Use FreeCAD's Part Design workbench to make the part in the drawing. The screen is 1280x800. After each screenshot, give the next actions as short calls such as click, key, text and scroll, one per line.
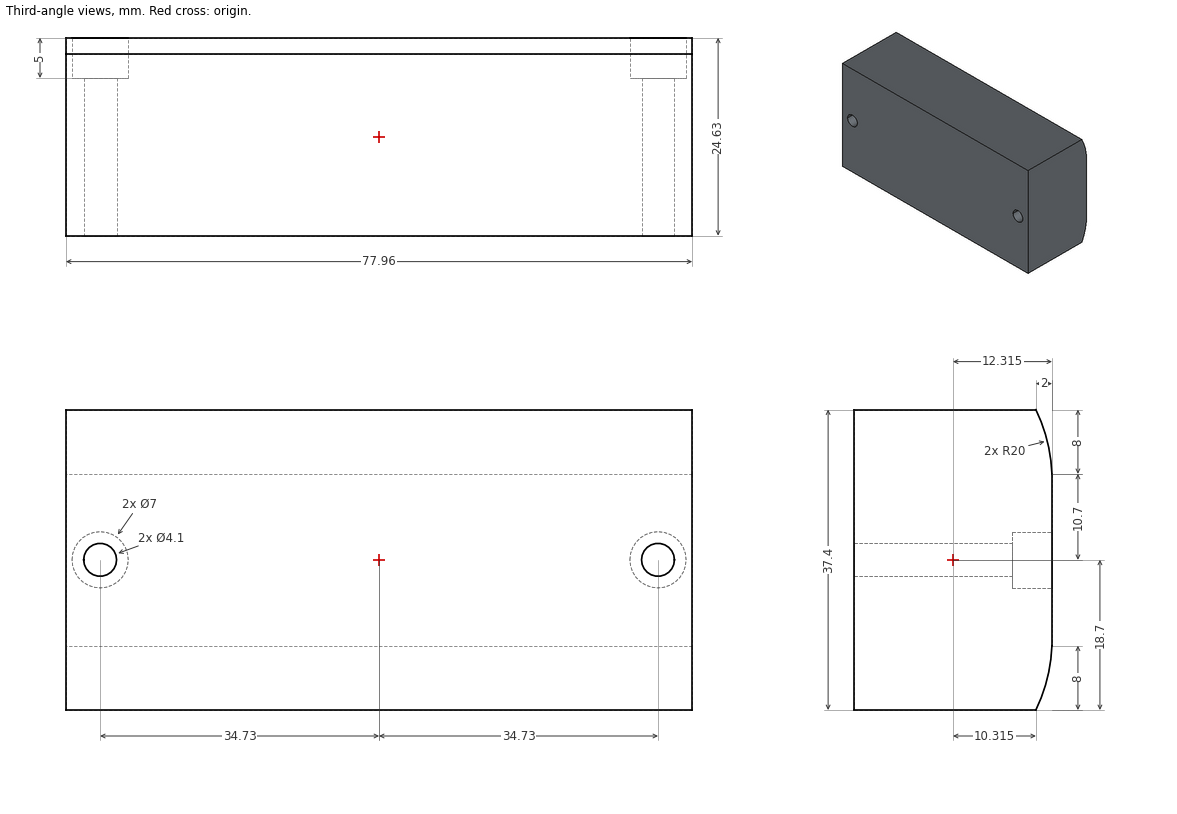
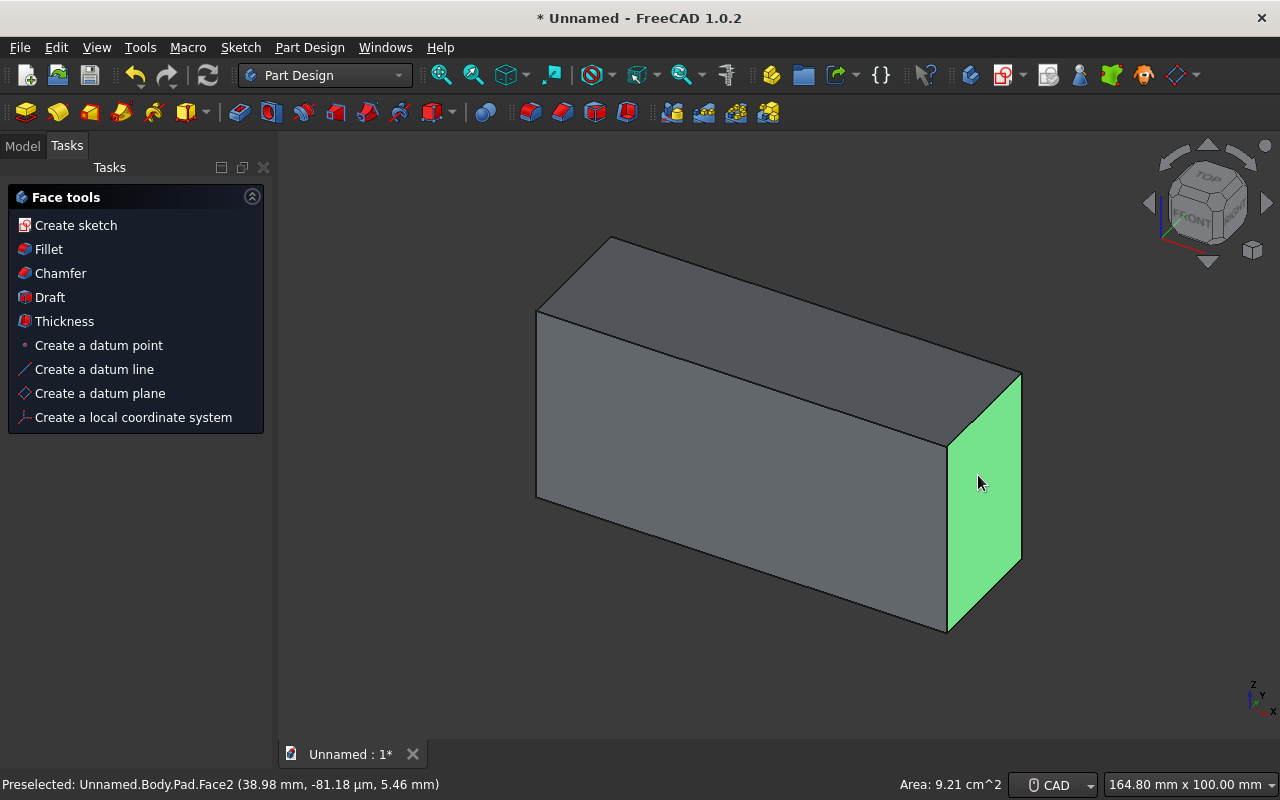
click(1004, 76)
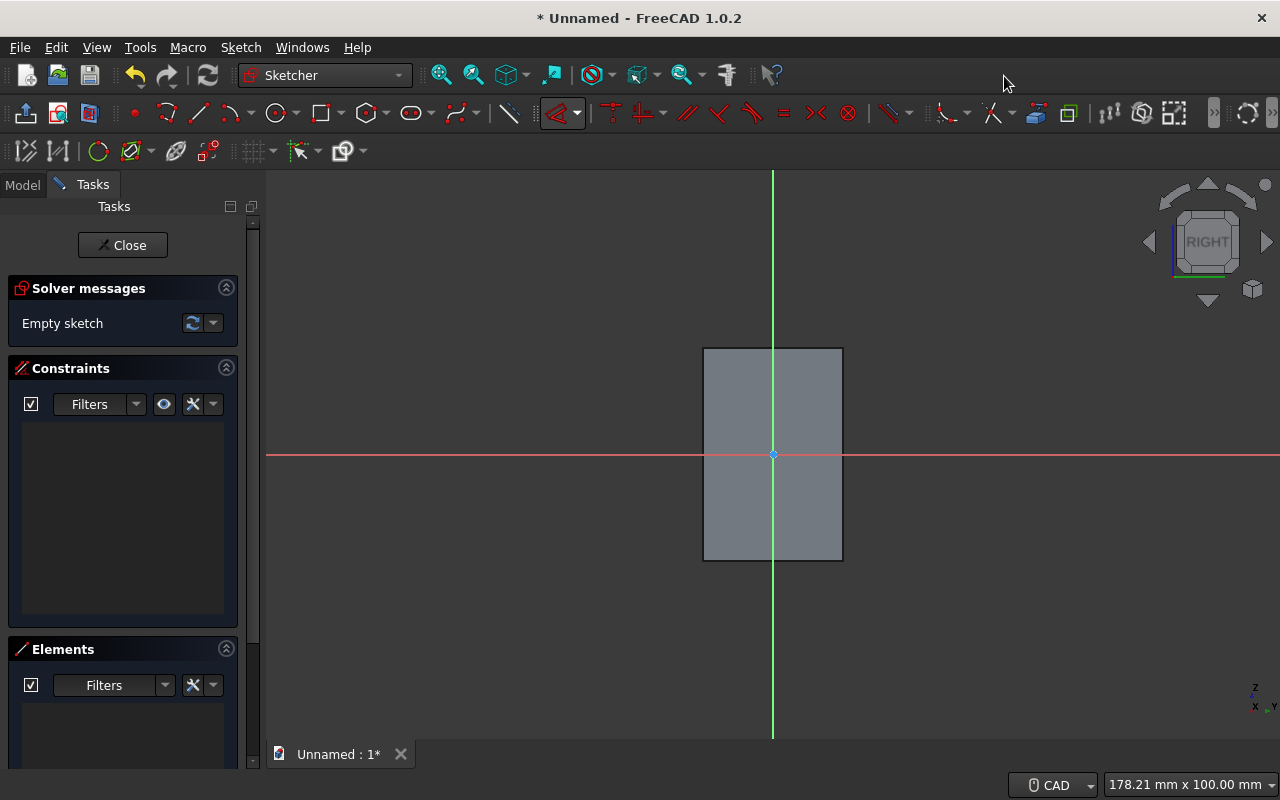
scroll(934, 454, up, 3)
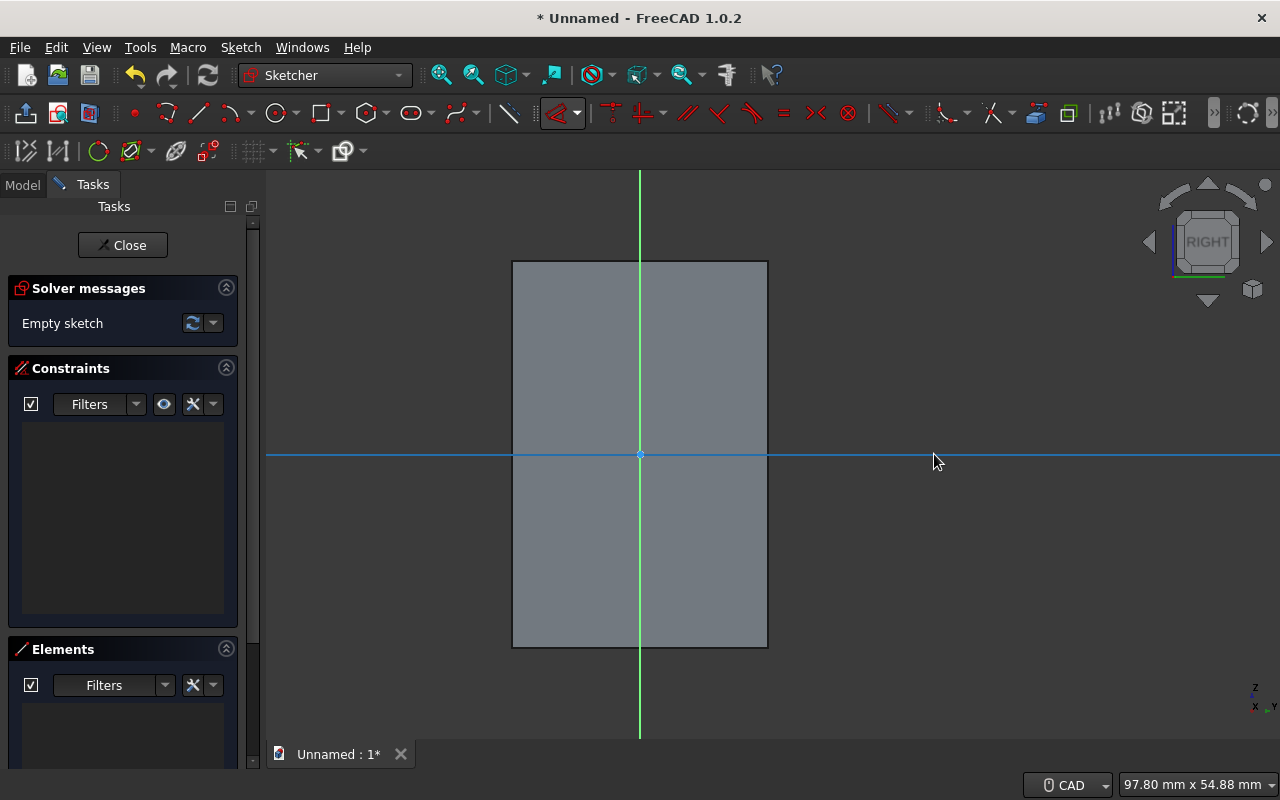
click(168, 114)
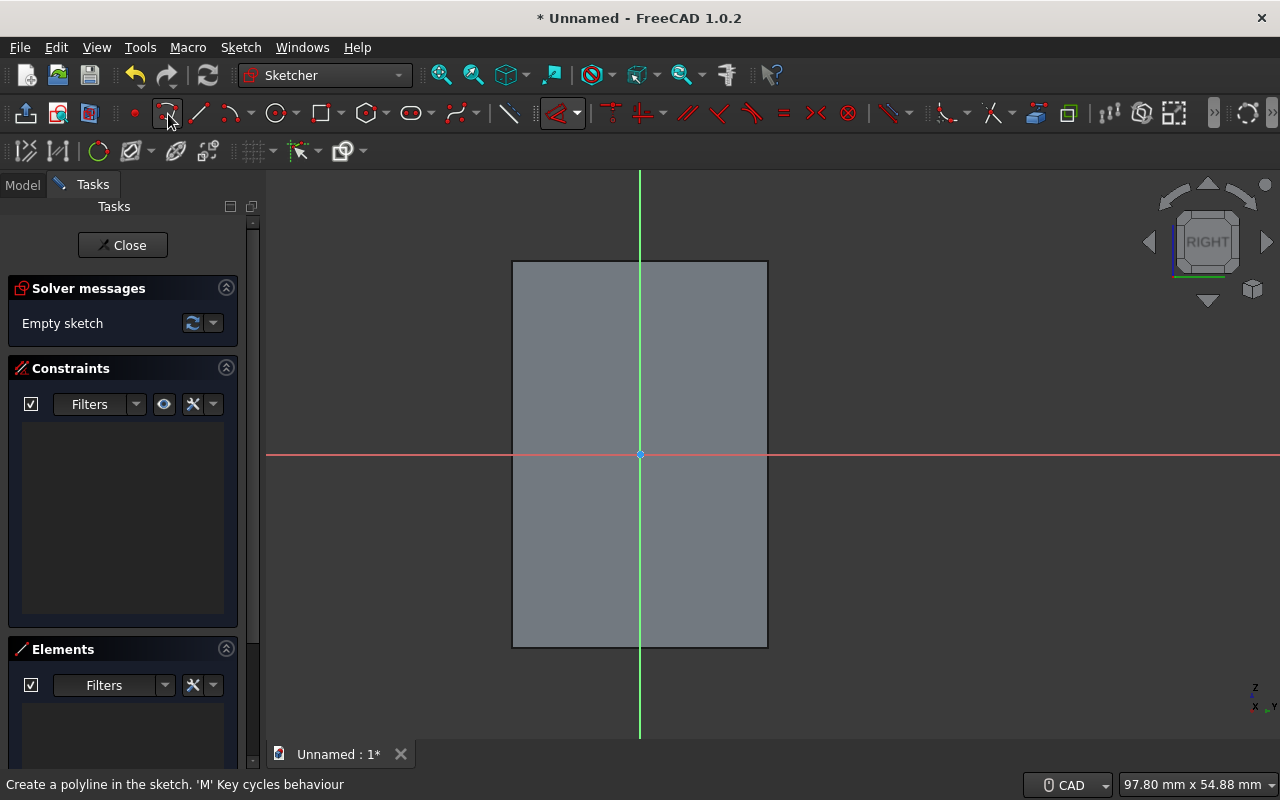
click(768, 344)
click(768, 261)
click(747, 261)
right_click(747, 261)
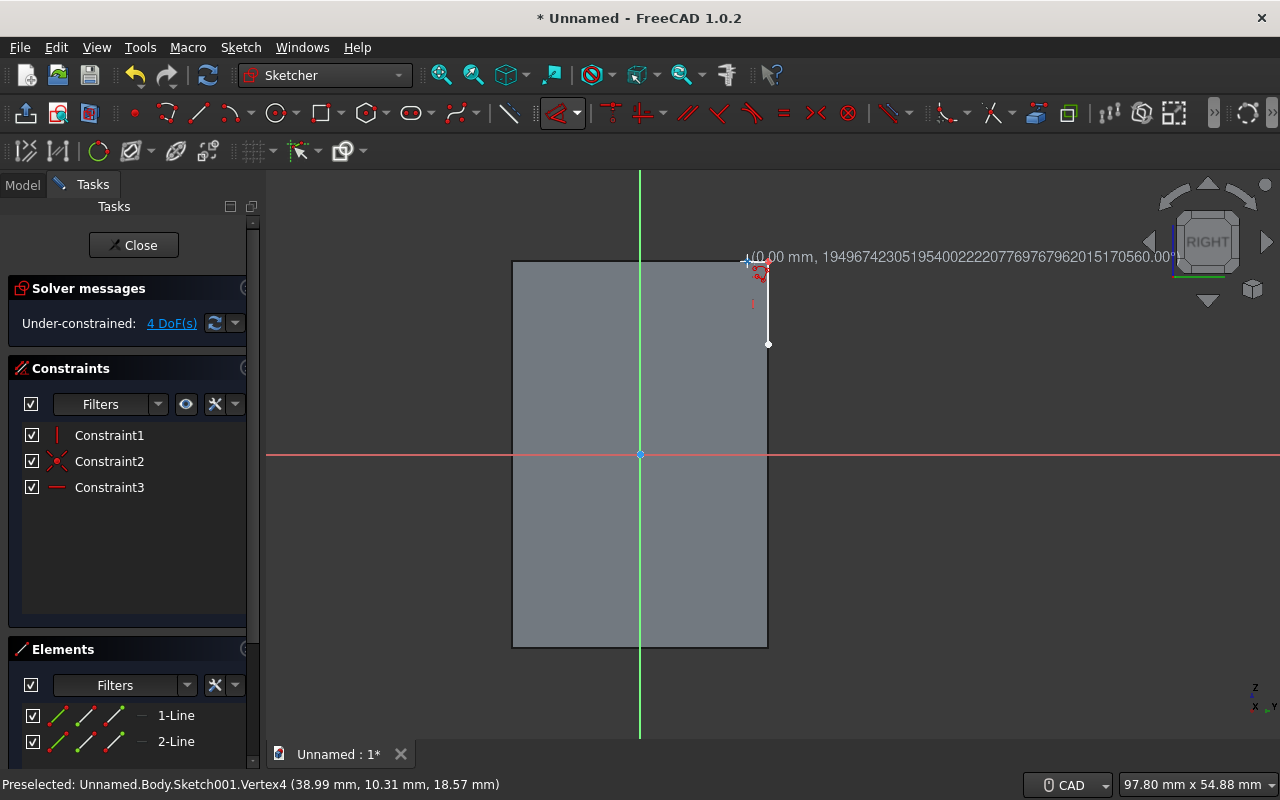
click(254, 114)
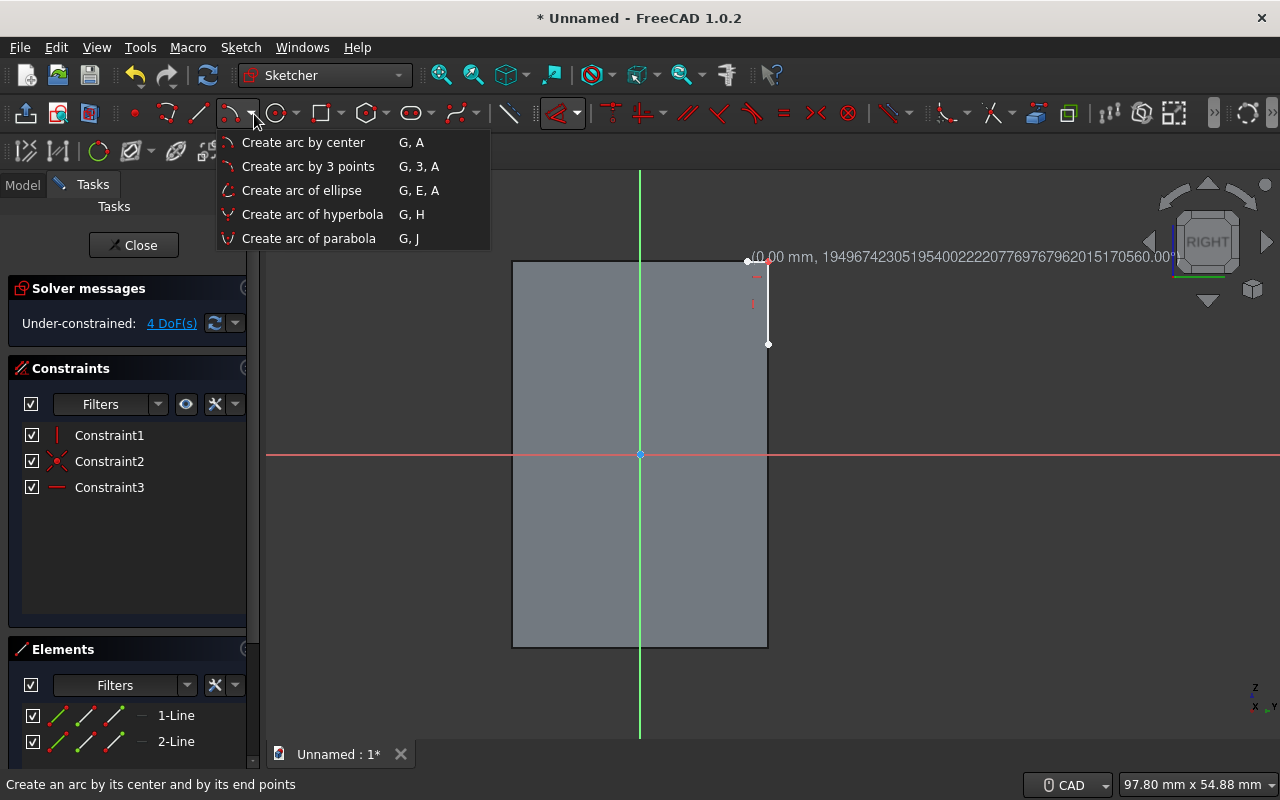
click(354, 166)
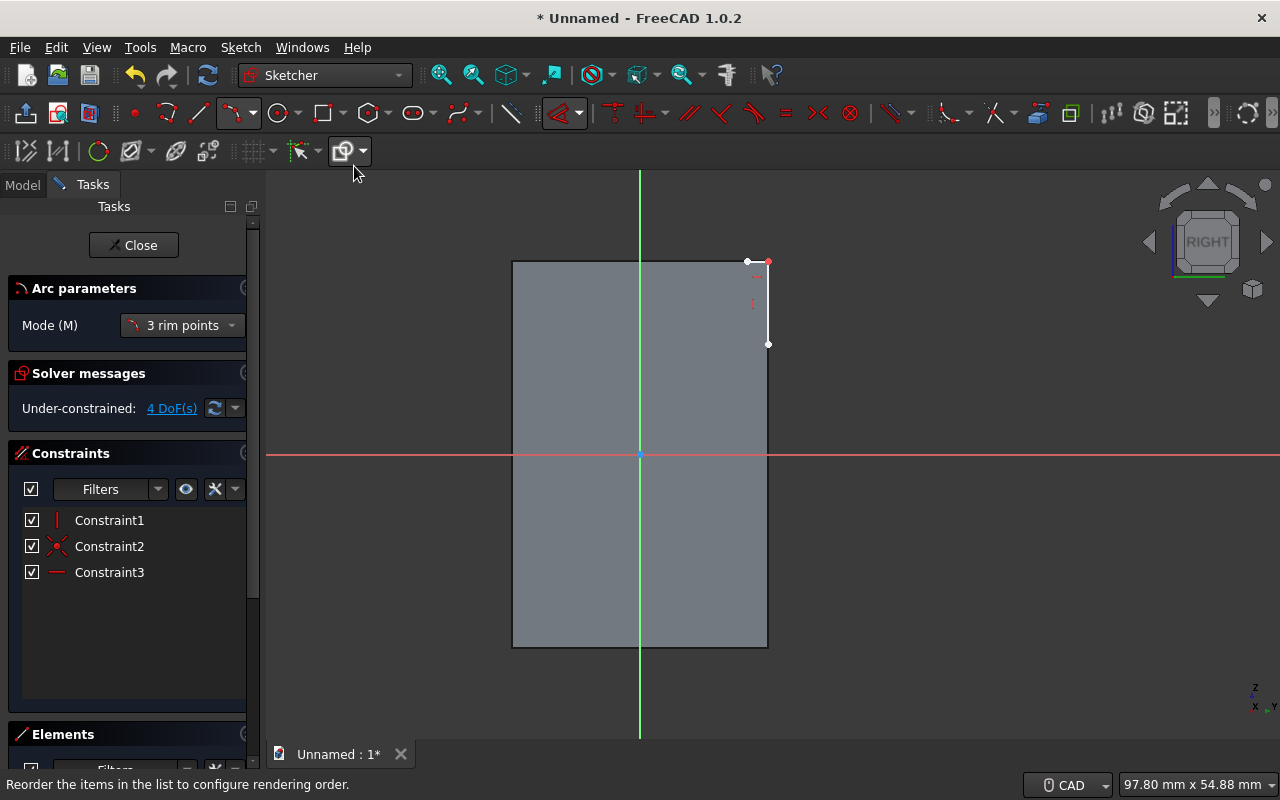
scroll(747, 261, up, 3)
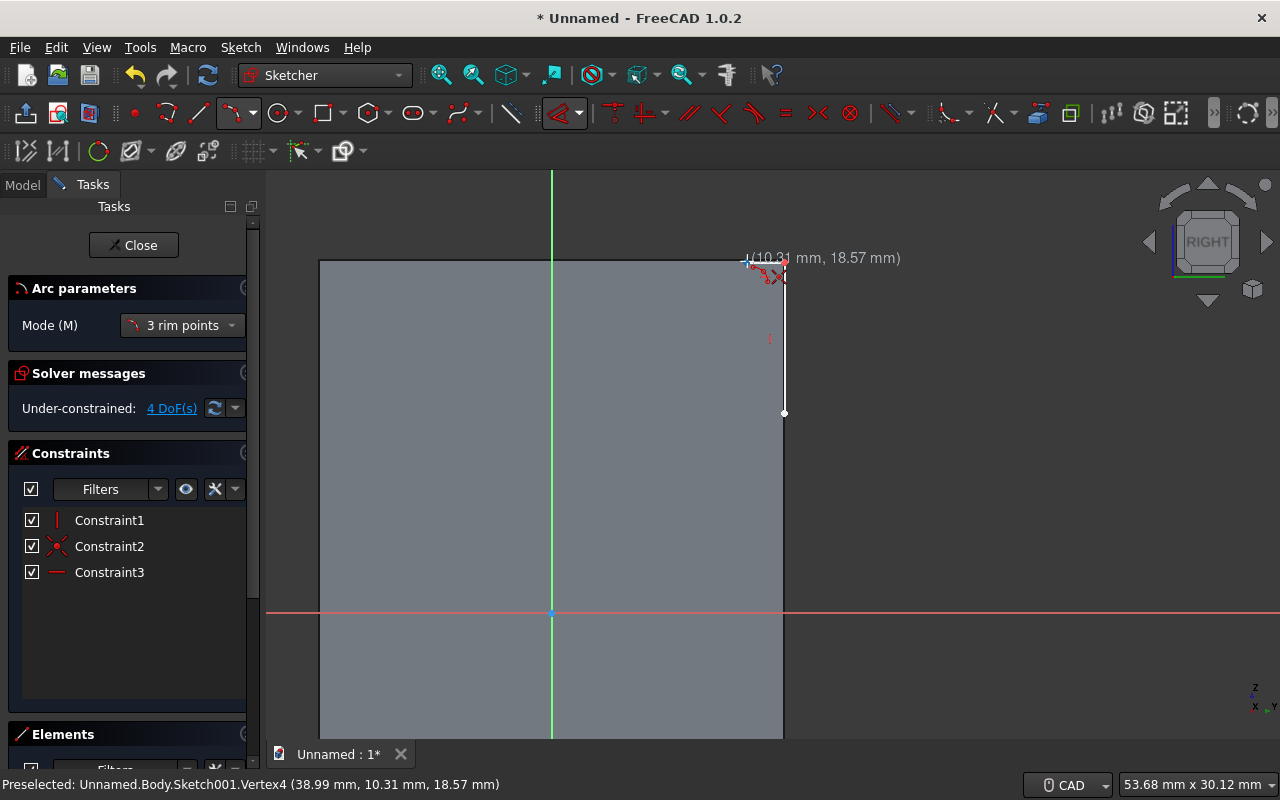
click(747, 263)
click(785, 414)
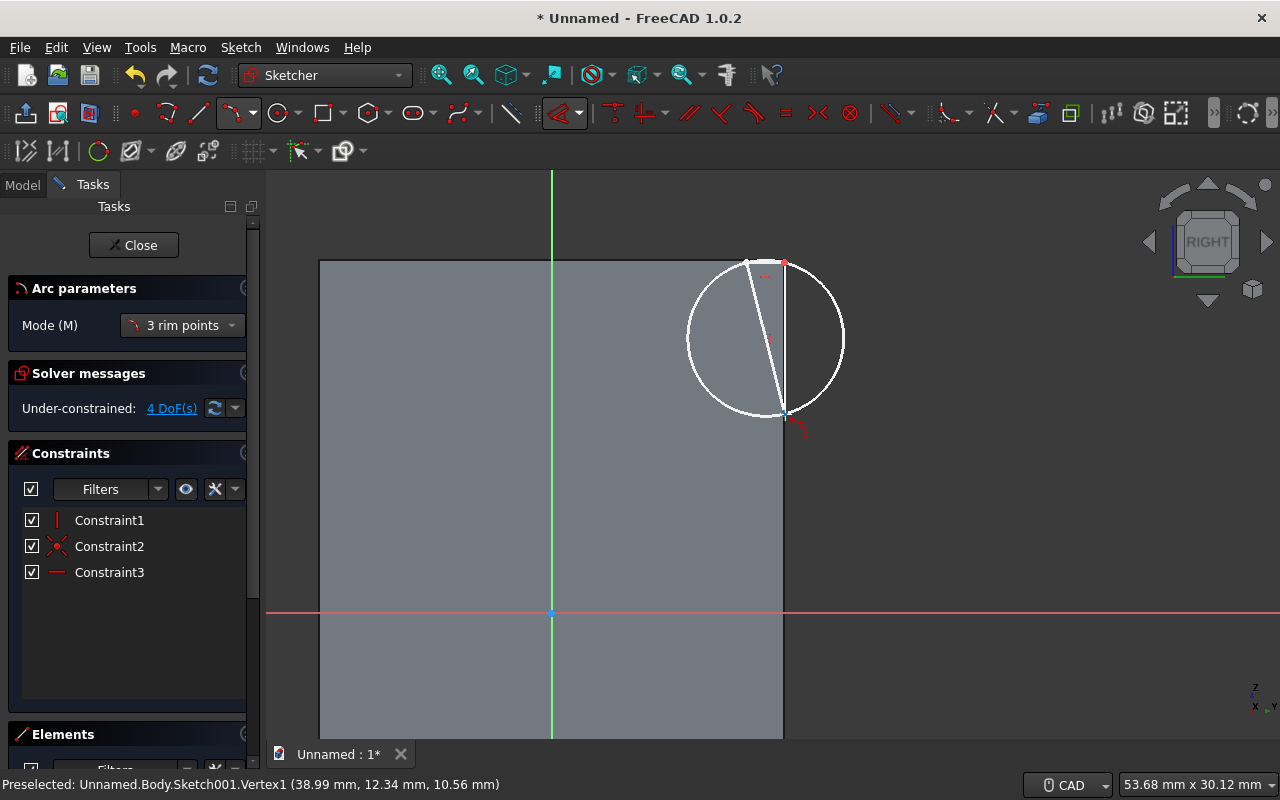
scroll(773, 334, up, 4)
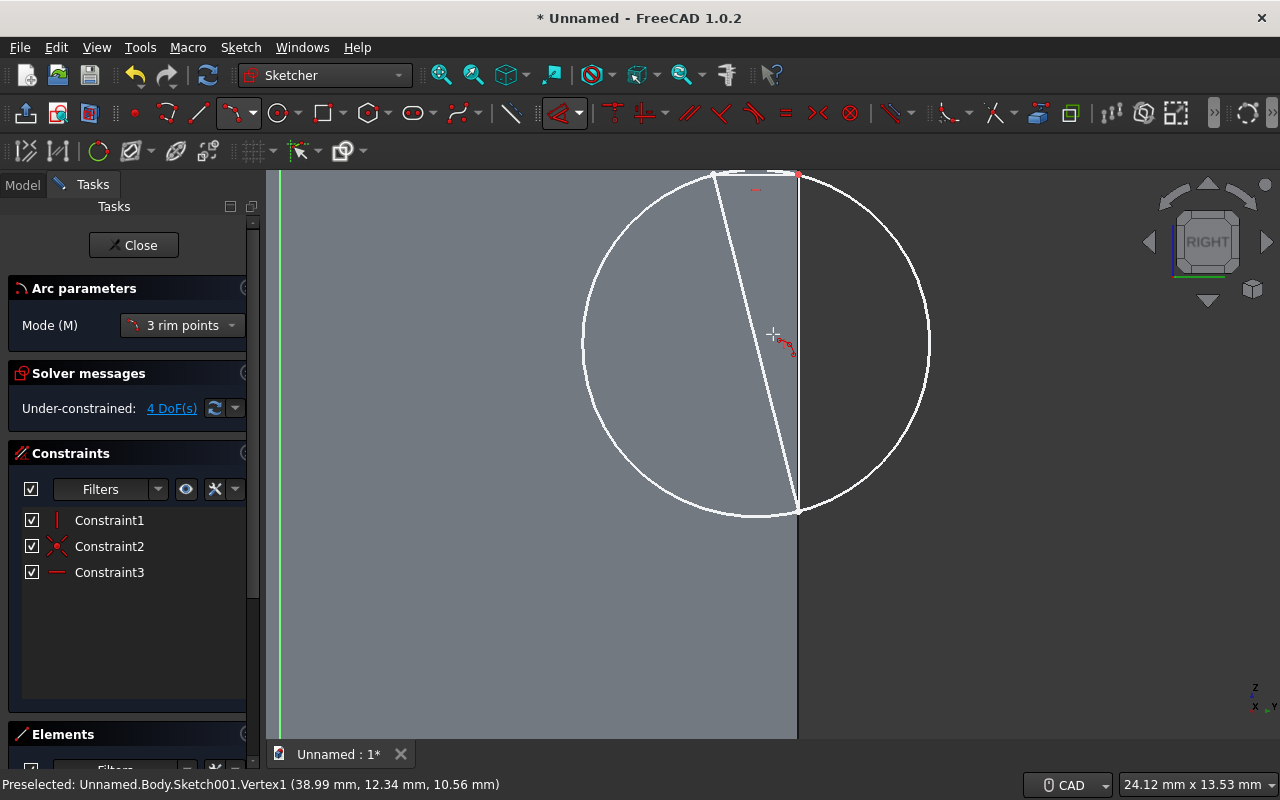
click(773, 333)